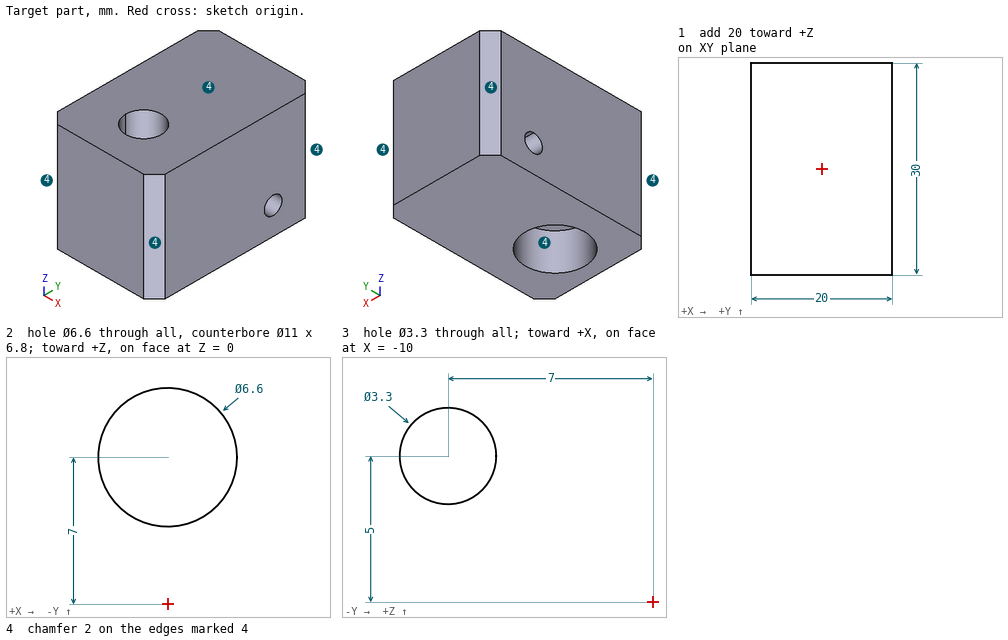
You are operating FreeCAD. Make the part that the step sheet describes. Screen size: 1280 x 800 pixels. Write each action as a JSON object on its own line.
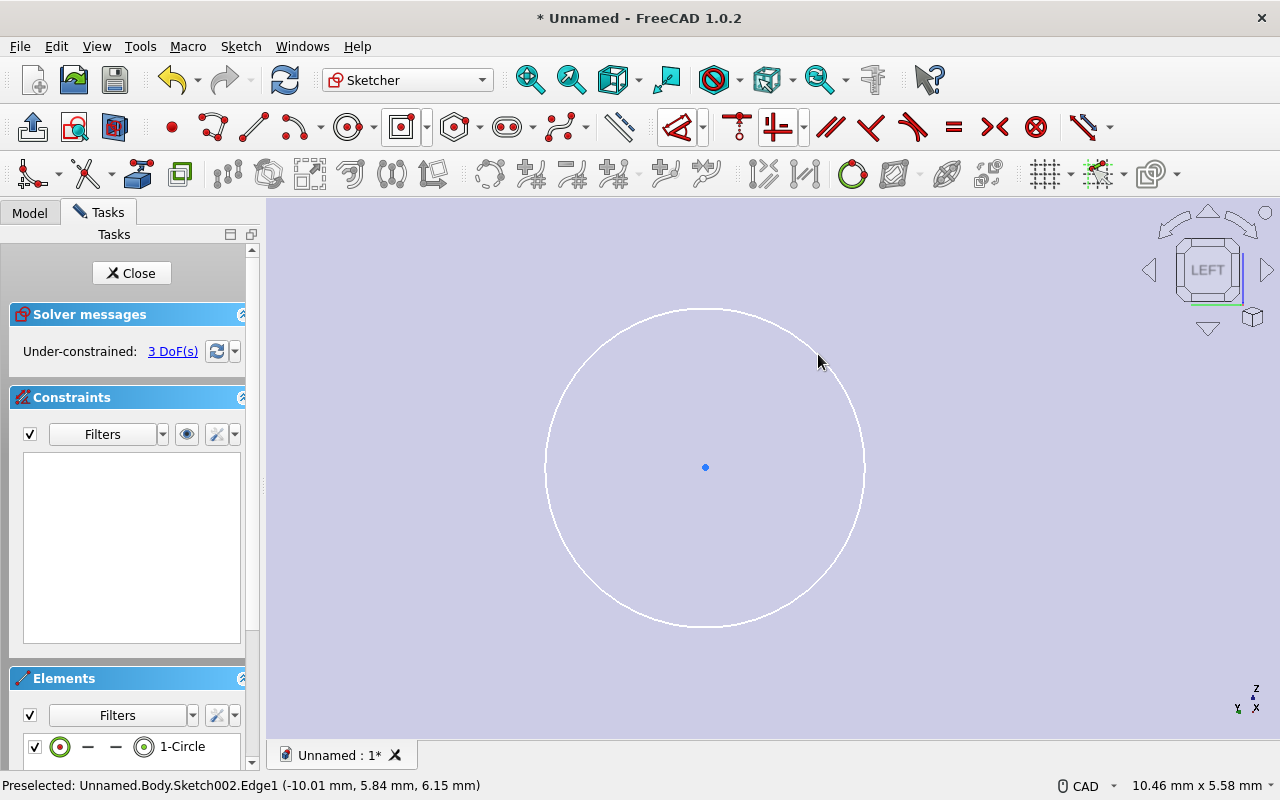
{"action": "left_click", "coordinate": [818, 355]}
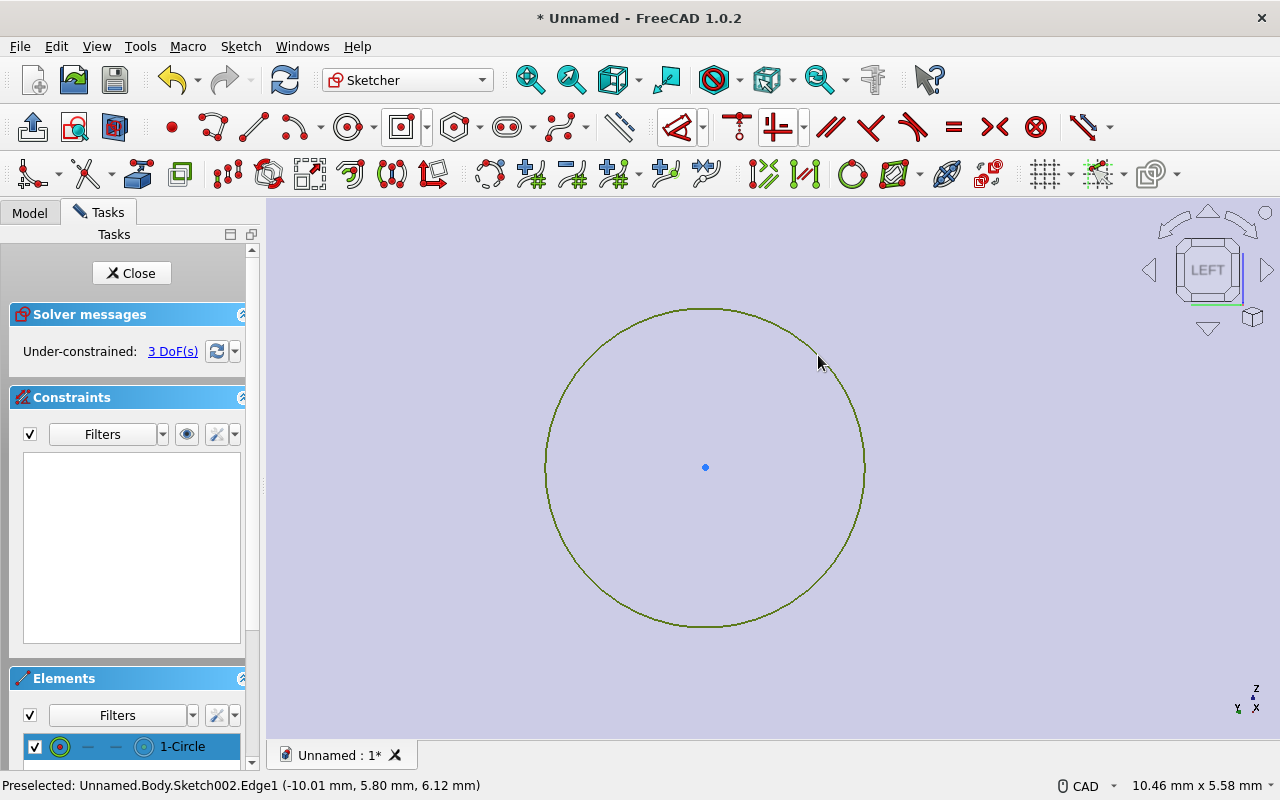
{"action": "key", "text": "k o"}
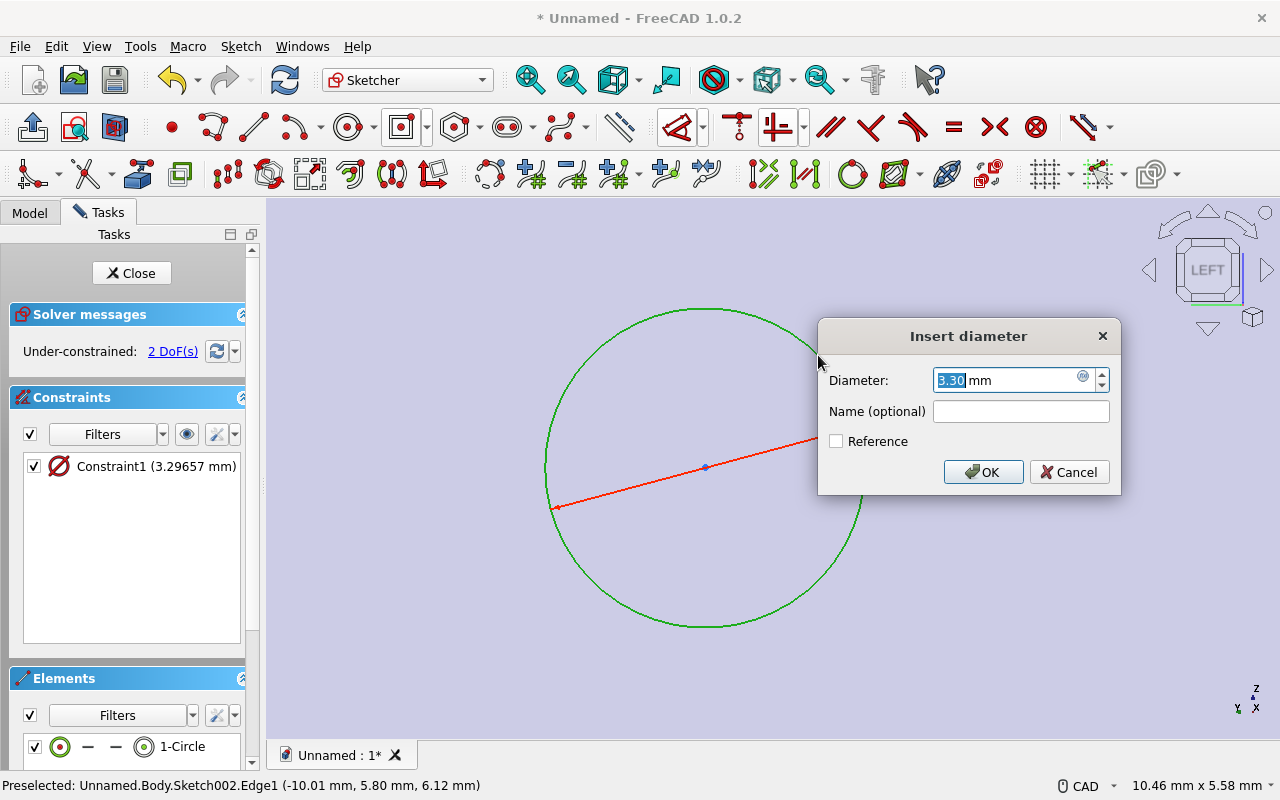
{"action": "type", "text": "3.3"}
{"action": "key", "text": "Return"}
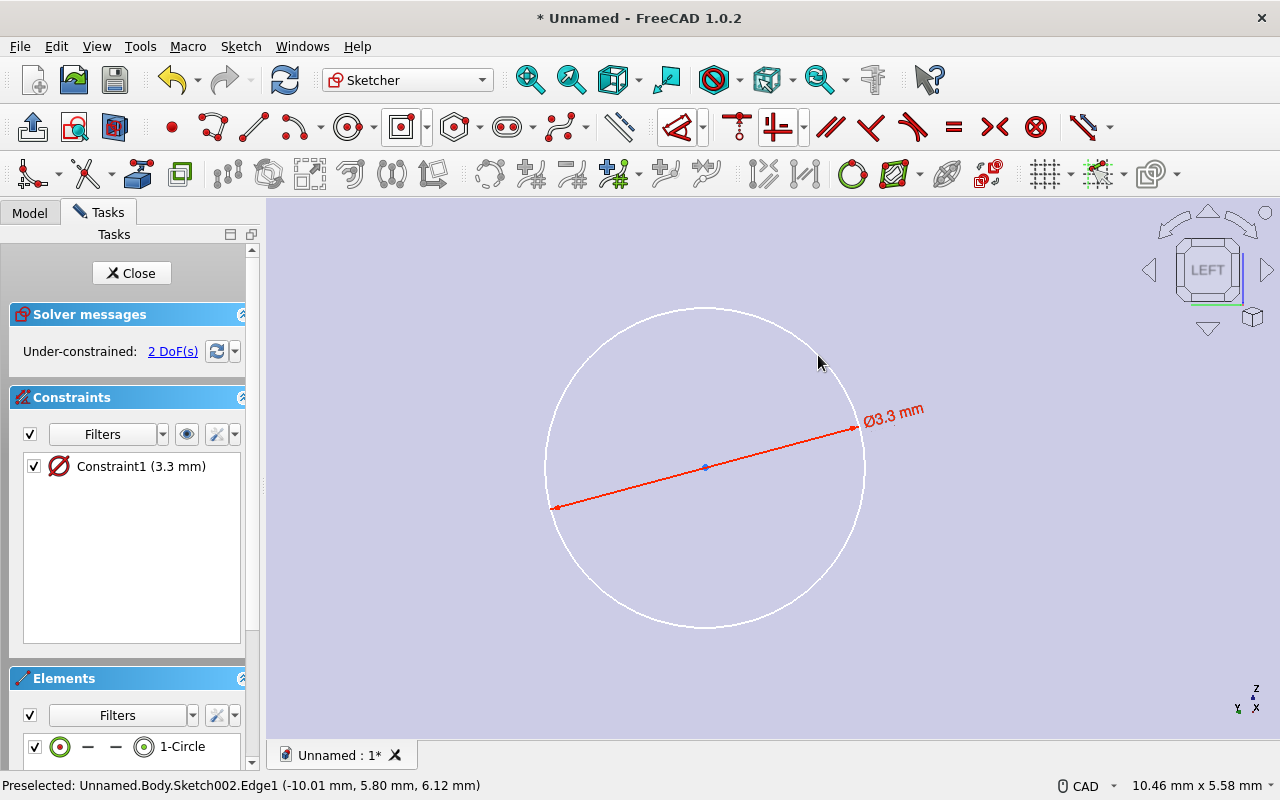
{"action": "left_click", "coordinate": [705, 468]}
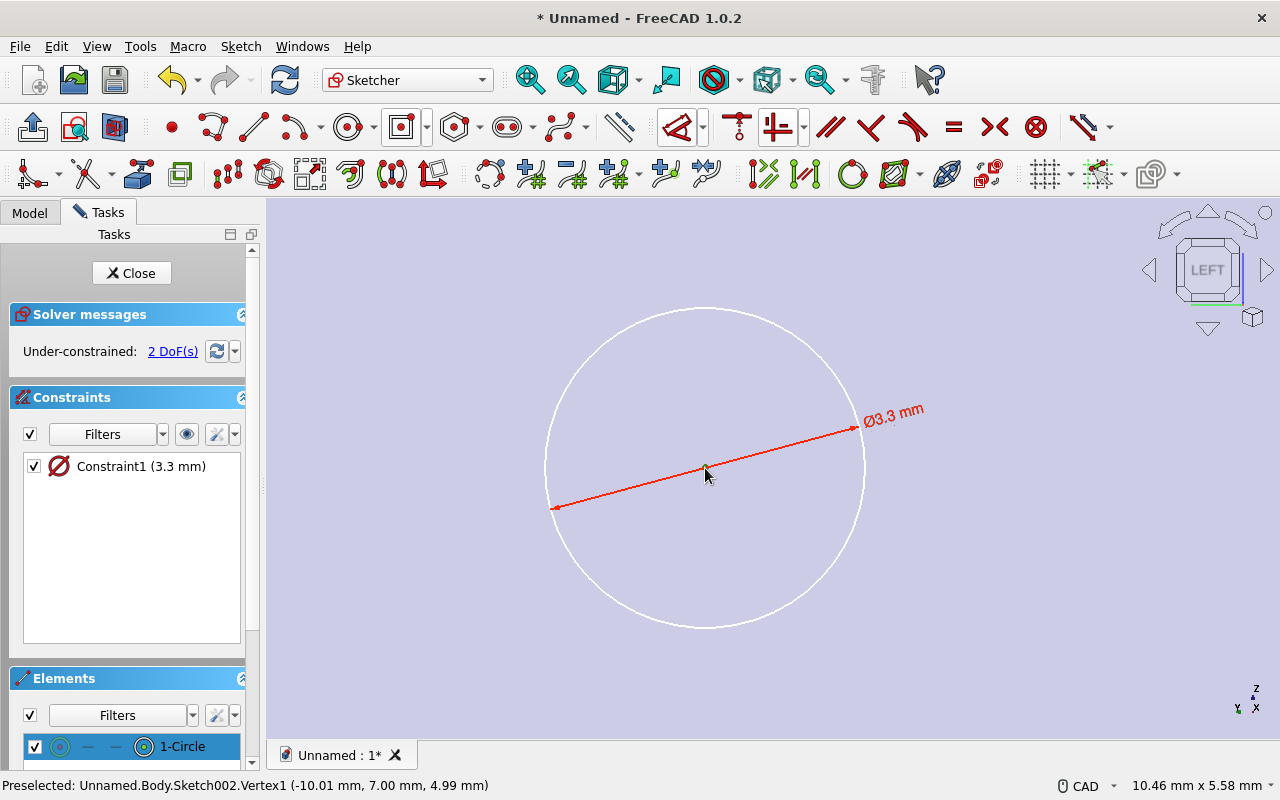
{"action": "key", "text": "l"}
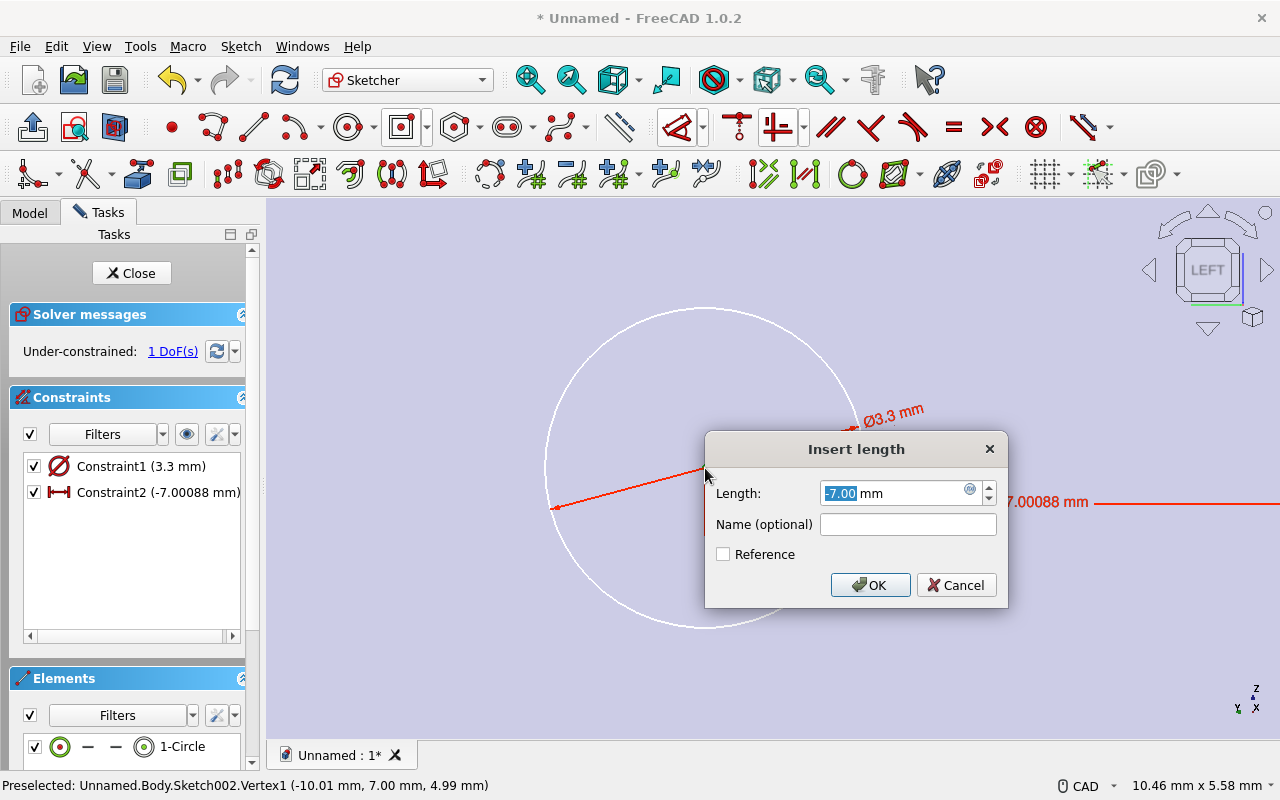
{"action": "type", "text": "-7"}
{"action": "key", "text": "Return"}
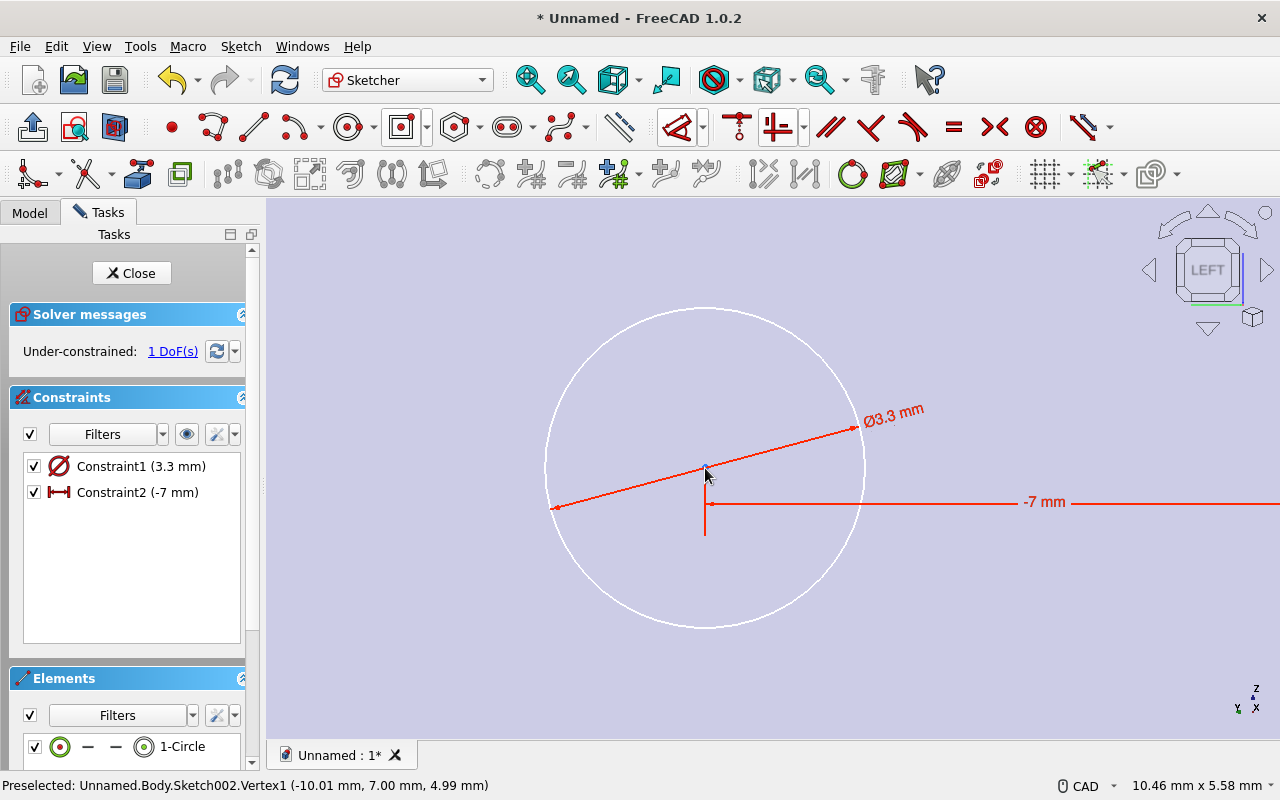
{"action": "left_click", "coordinate": [705, 468]}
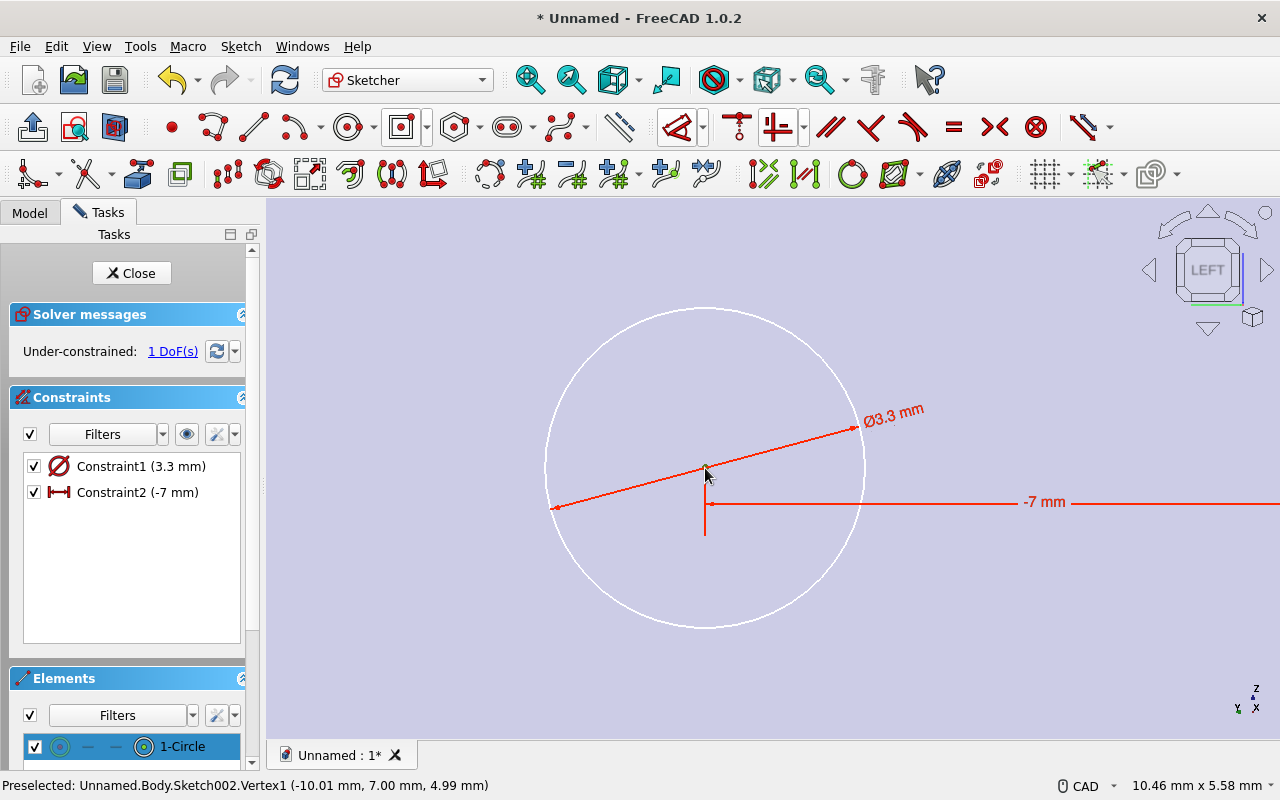
{"action": "key", "text": "i"}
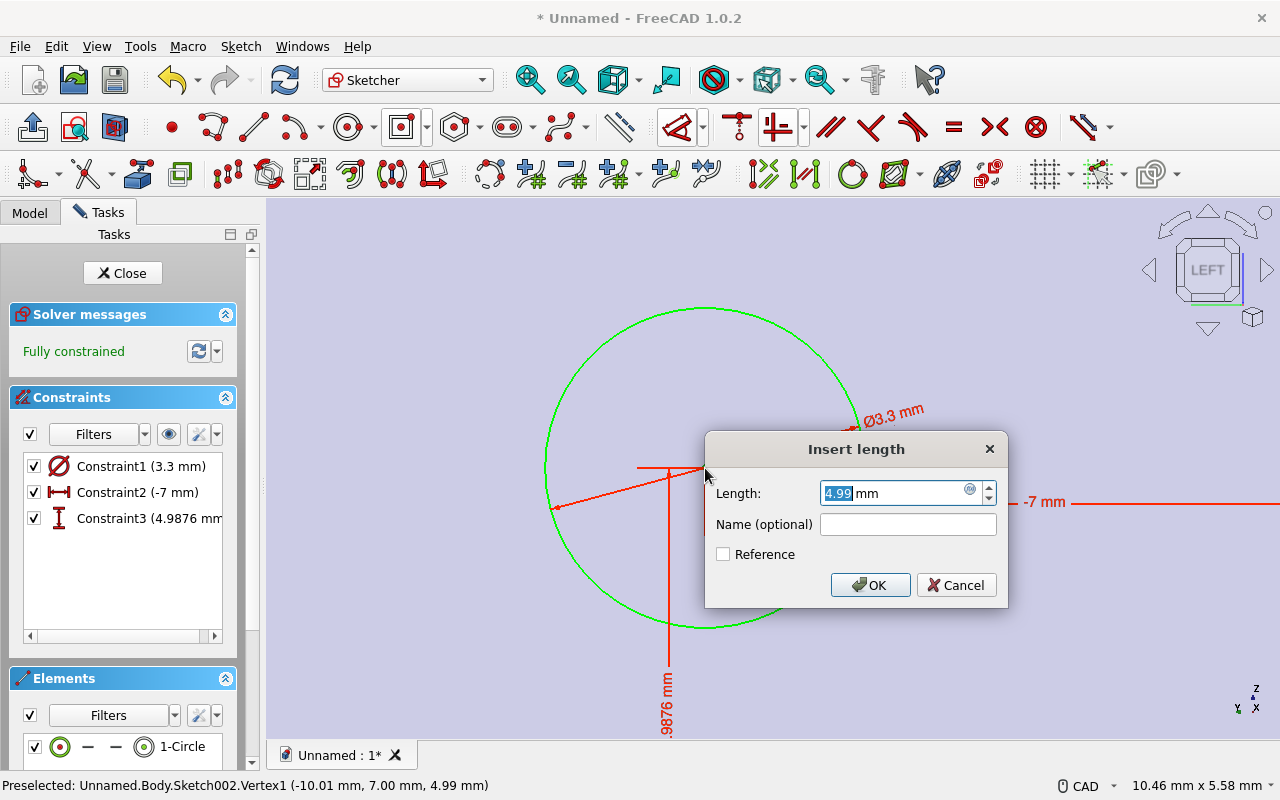
{"action": "type", "text": "5"}
{"action": "key", "text": "Return"}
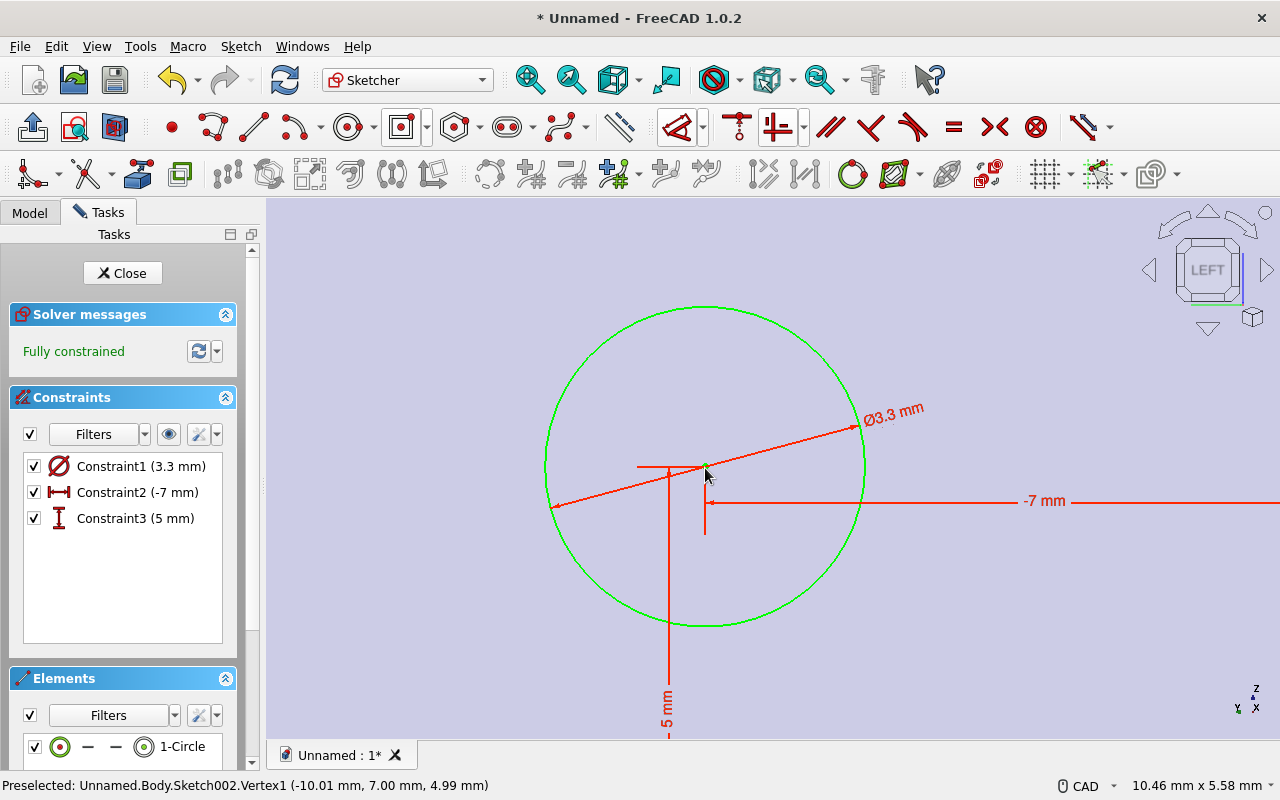
{"action": "left_click", "coordinate": [123, 273]}